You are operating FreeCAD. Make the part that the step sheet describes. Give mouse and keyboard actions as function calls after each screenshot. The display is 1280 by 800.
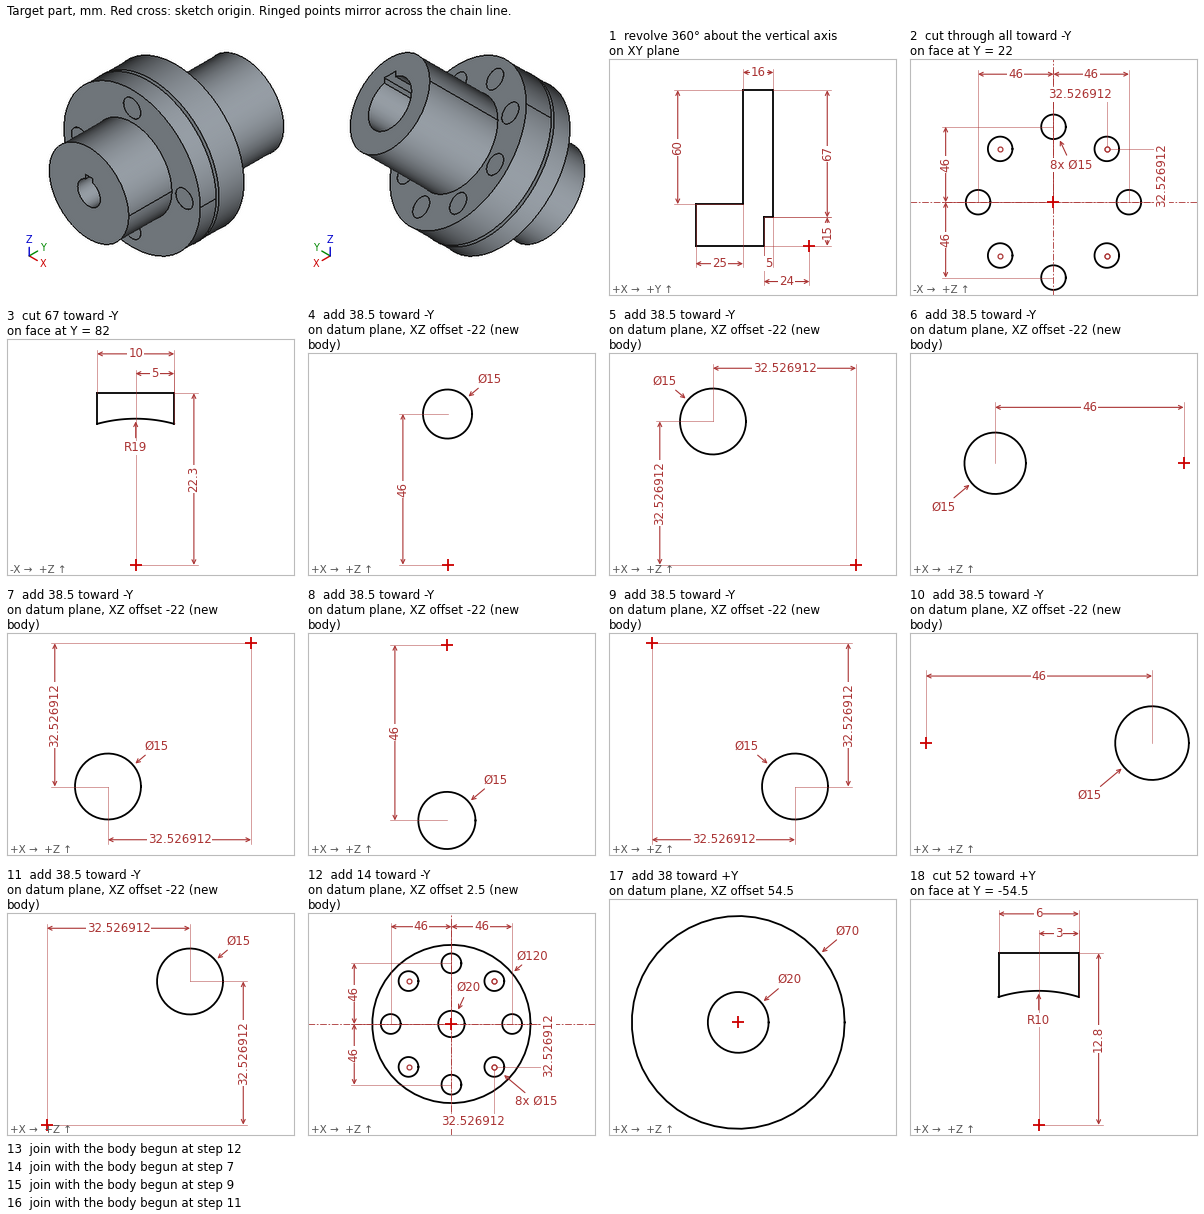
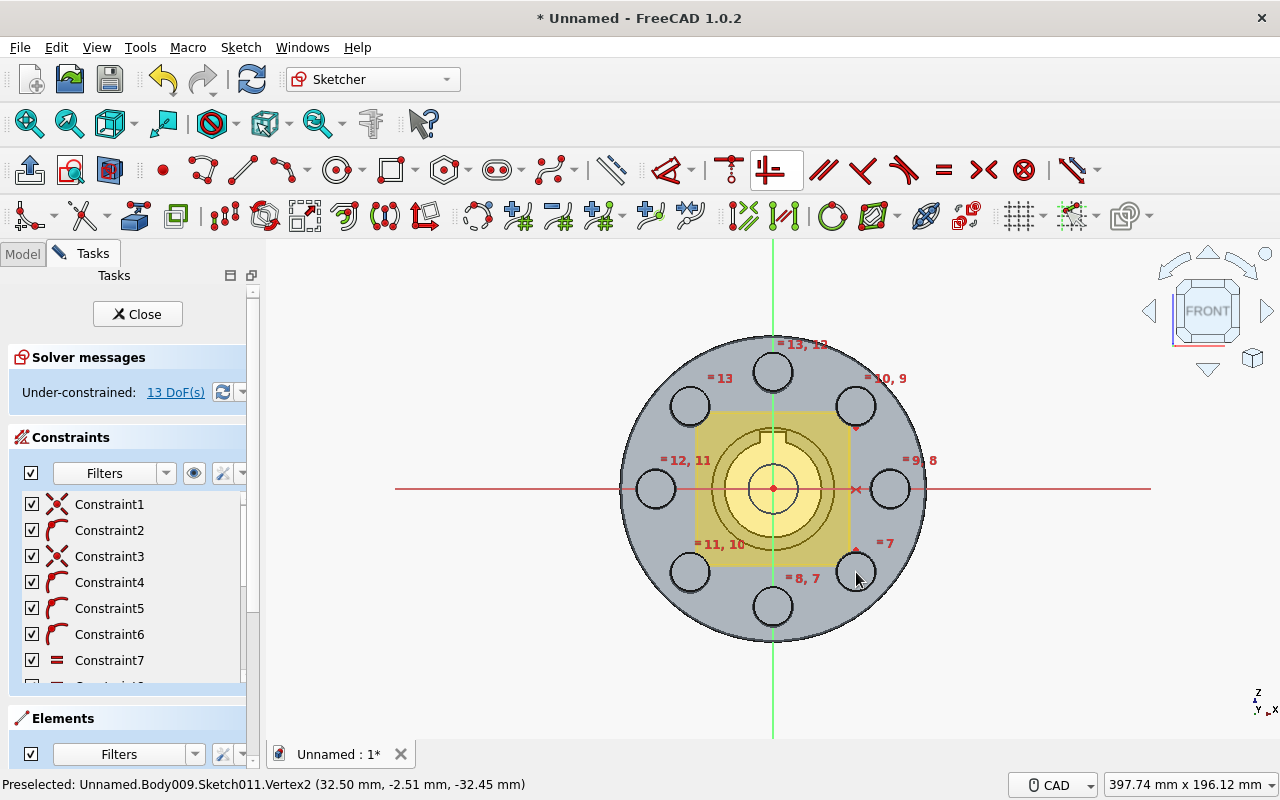
click(690, 573)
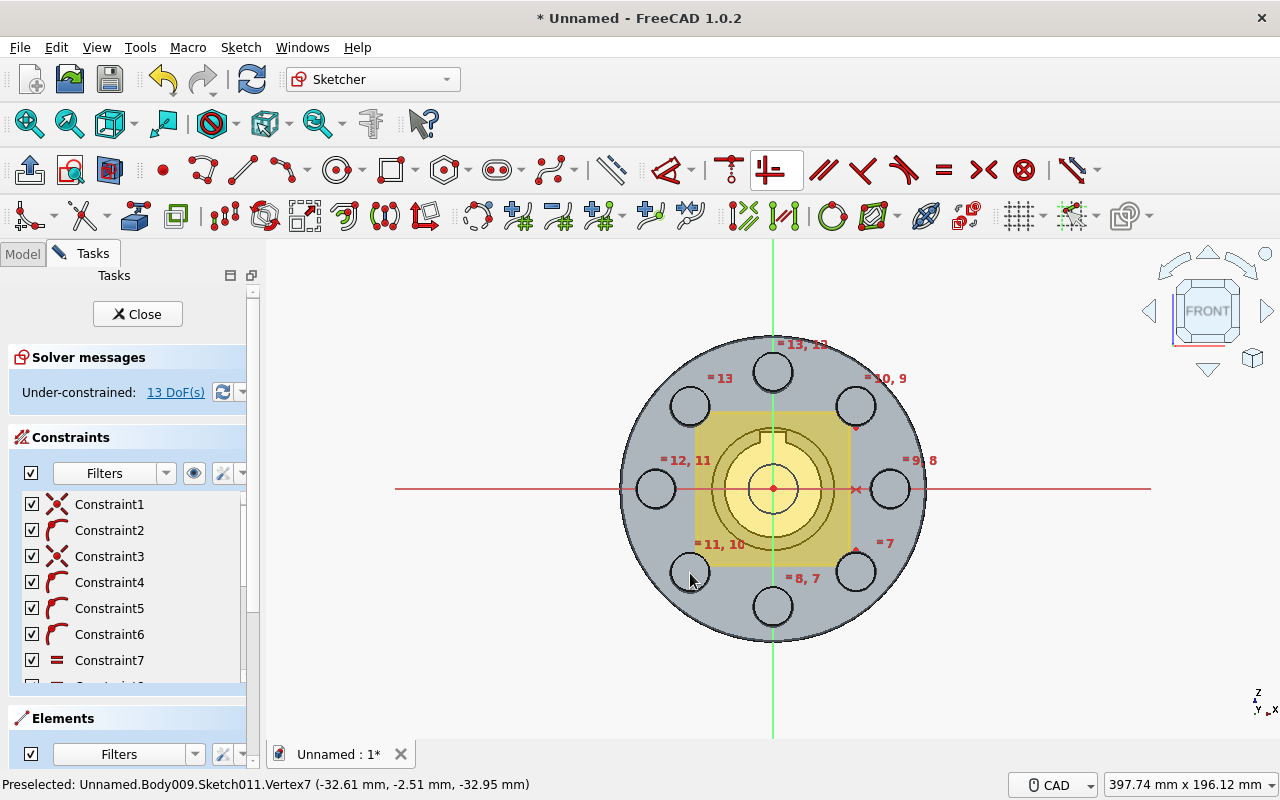
click(773, 679)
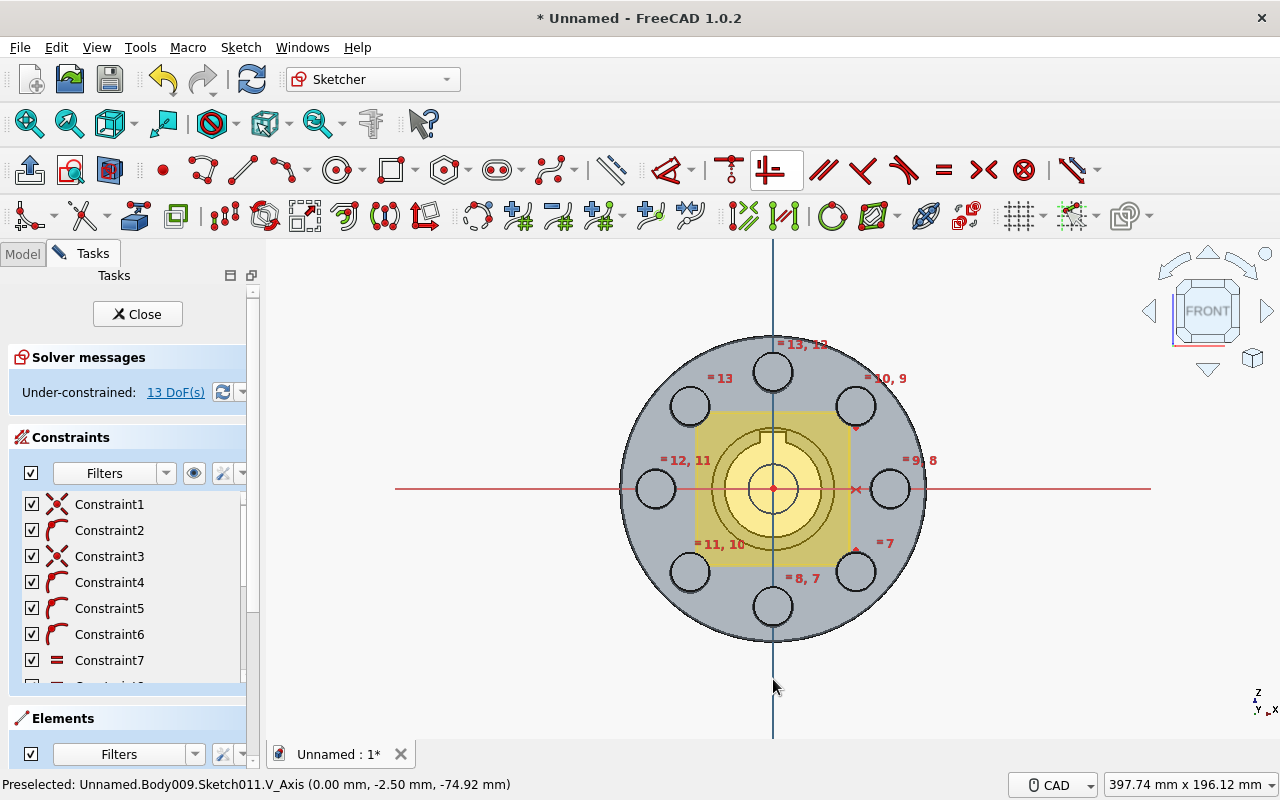
click(984, 170)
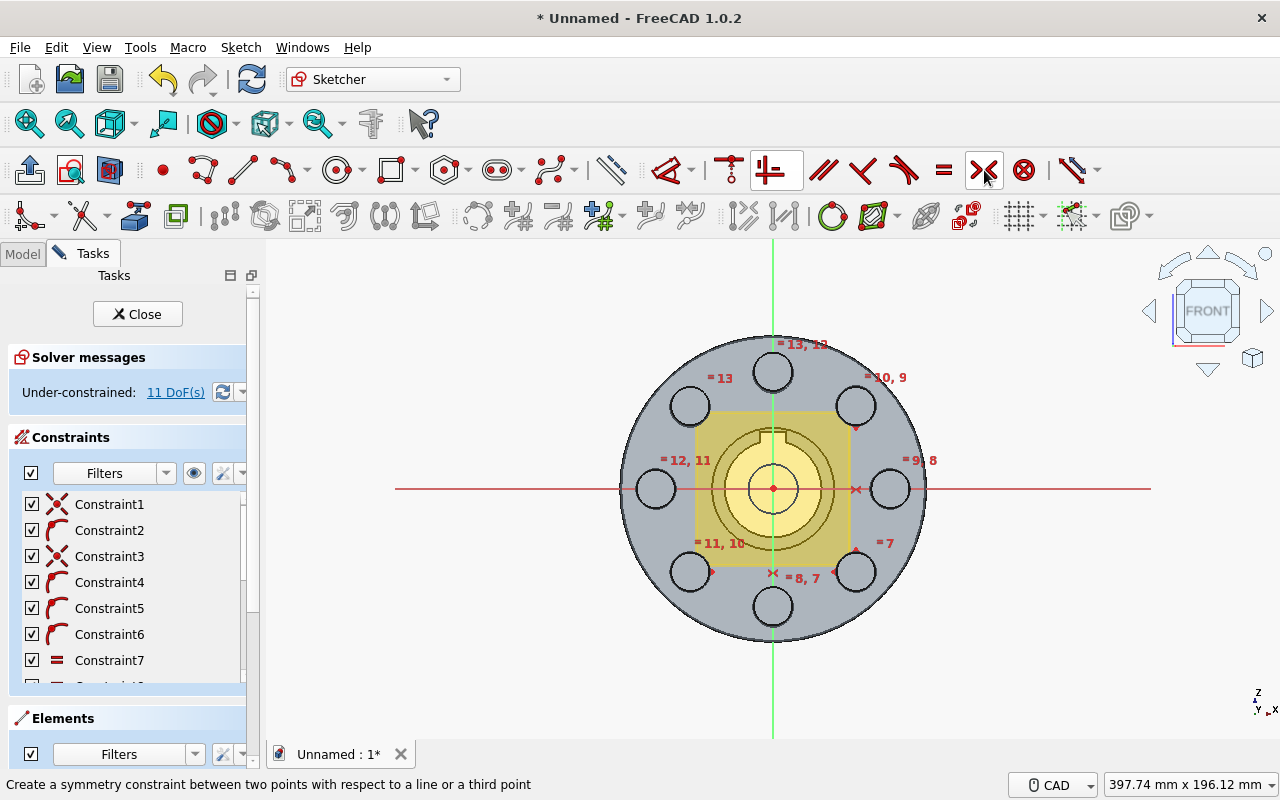
click(856, 406)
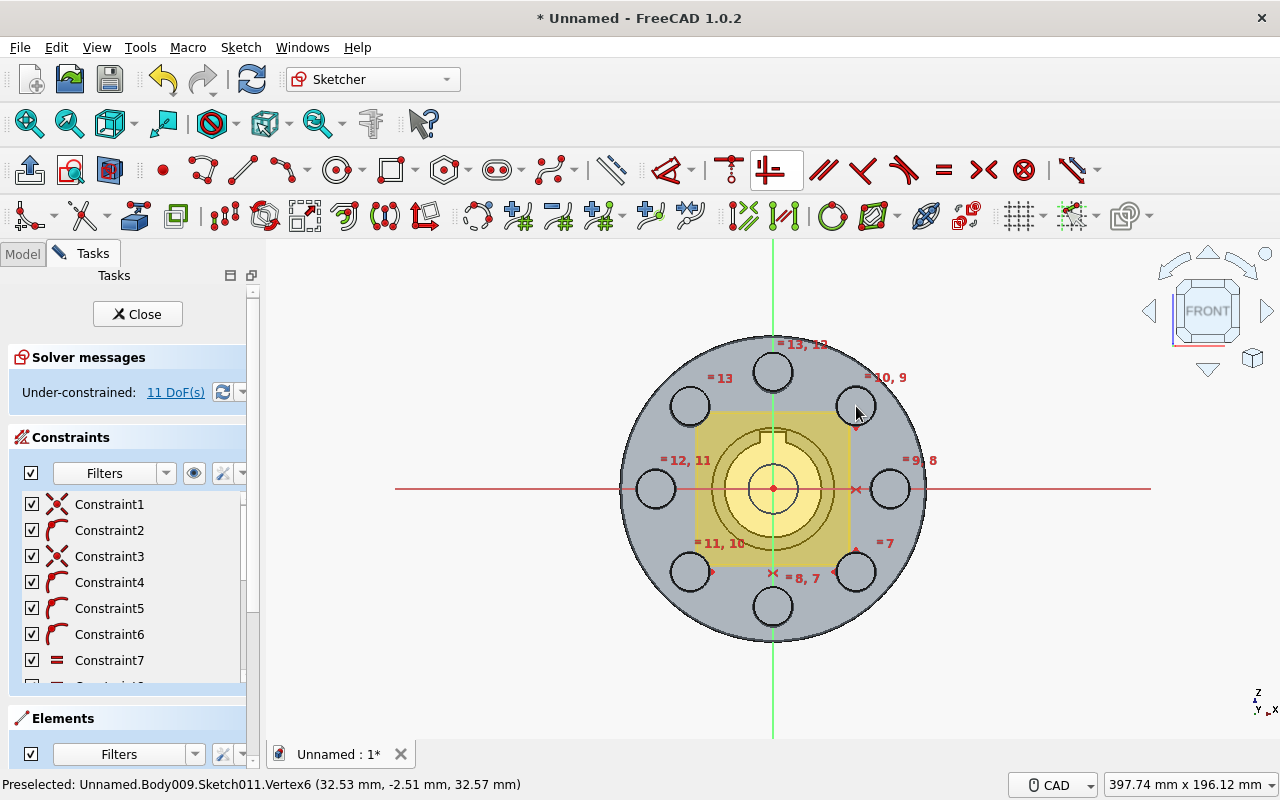
click(690, 407)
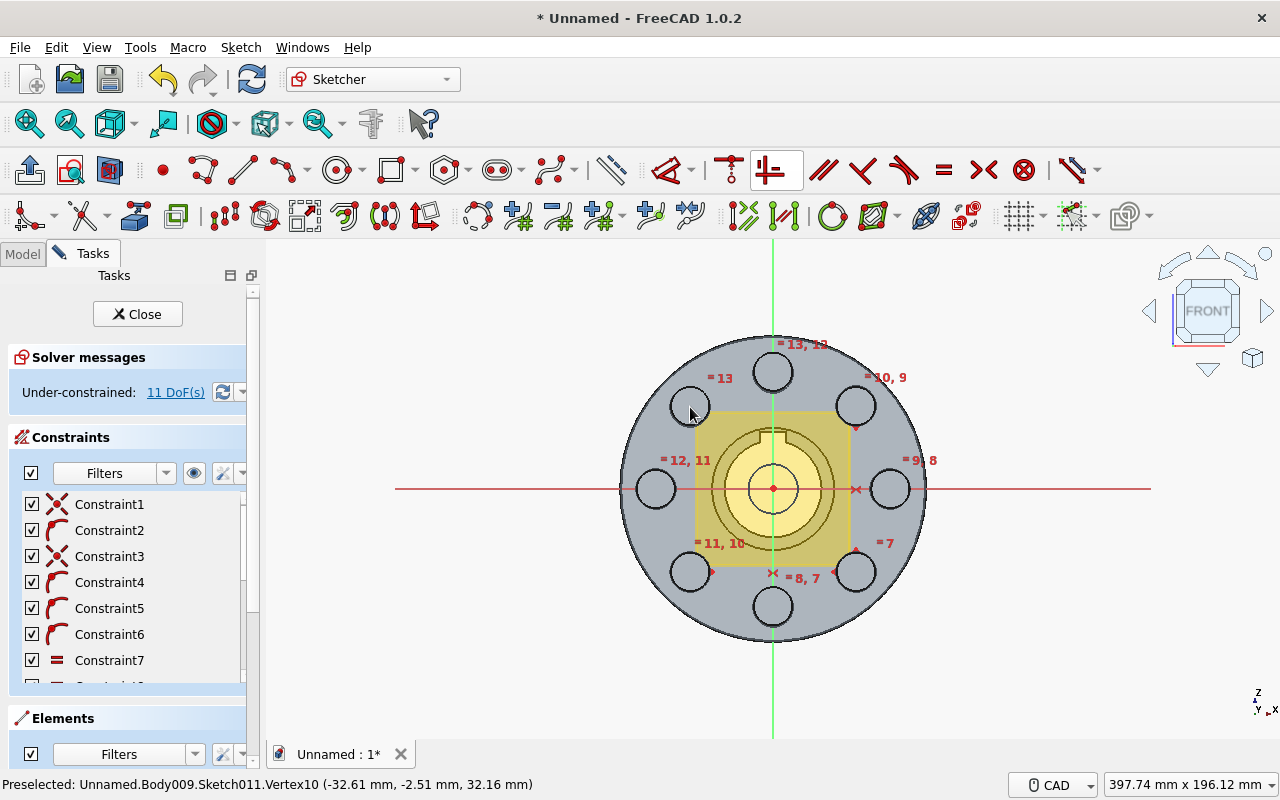
click(773, 679)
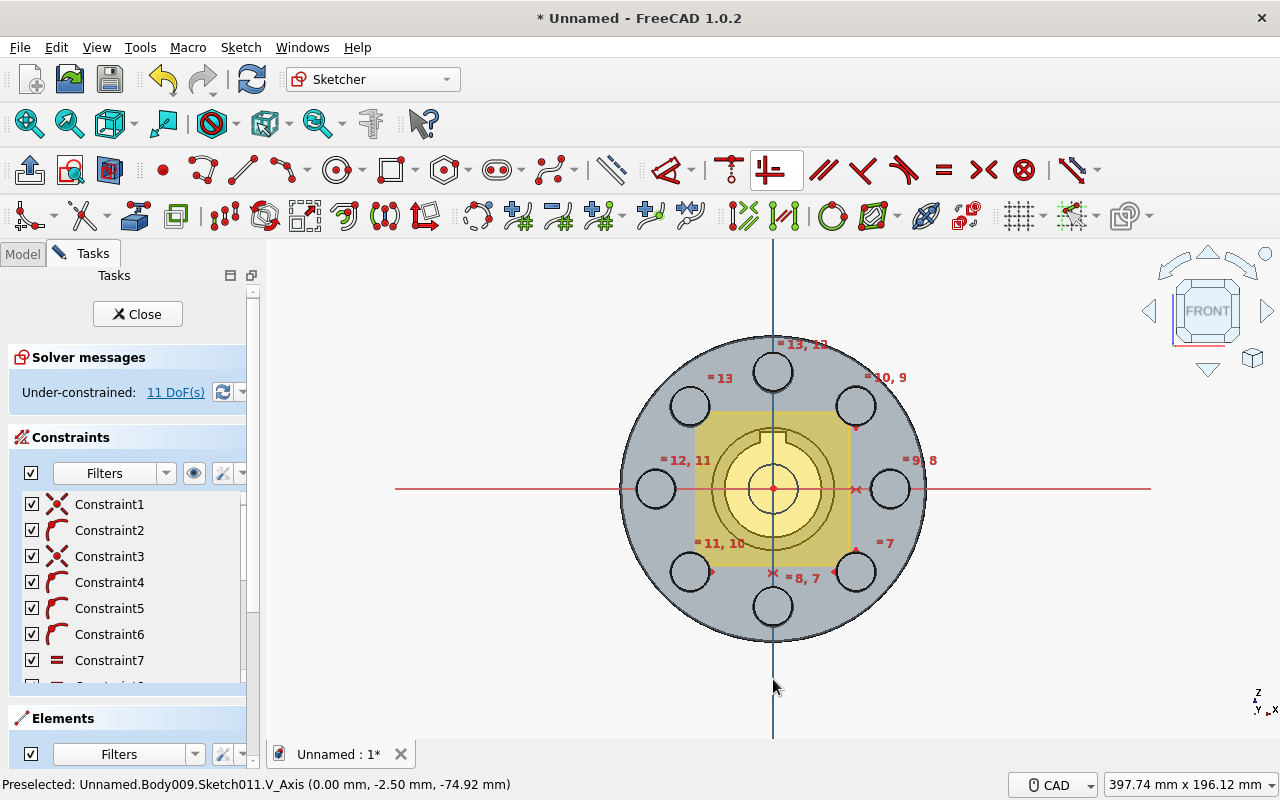
click(984, 170)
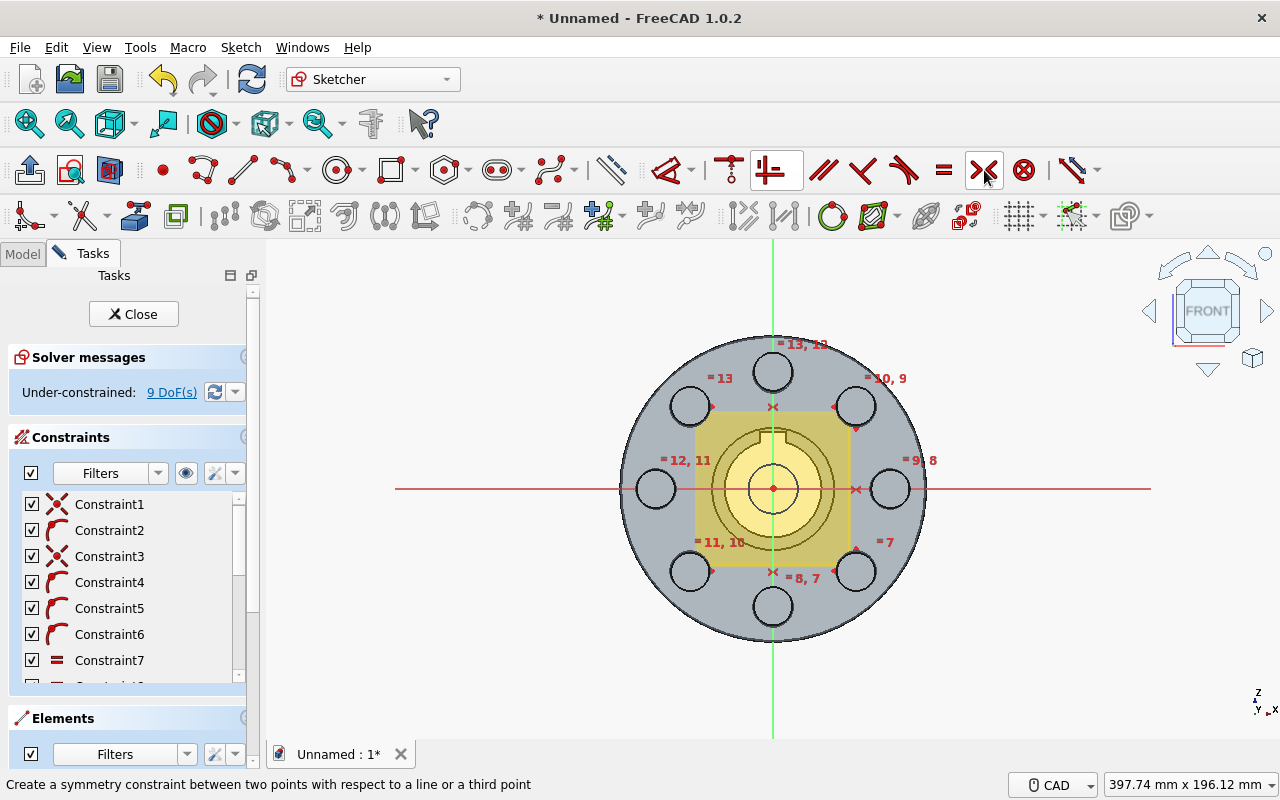
click(666, 170)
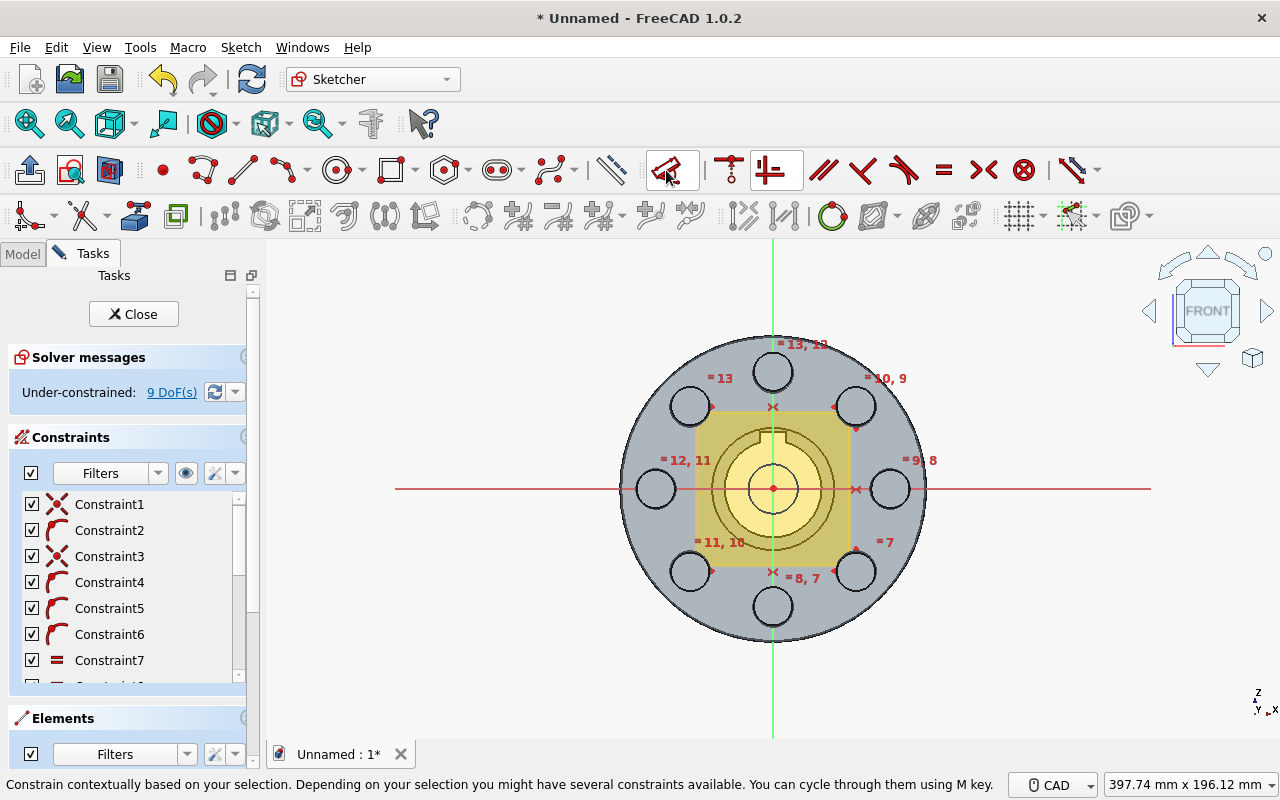
click(880, 381)
click(903, 358)